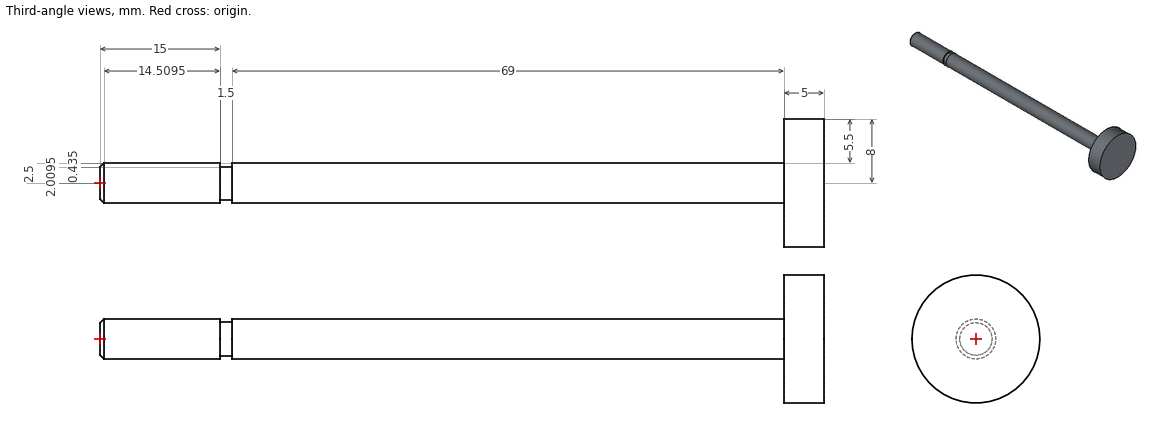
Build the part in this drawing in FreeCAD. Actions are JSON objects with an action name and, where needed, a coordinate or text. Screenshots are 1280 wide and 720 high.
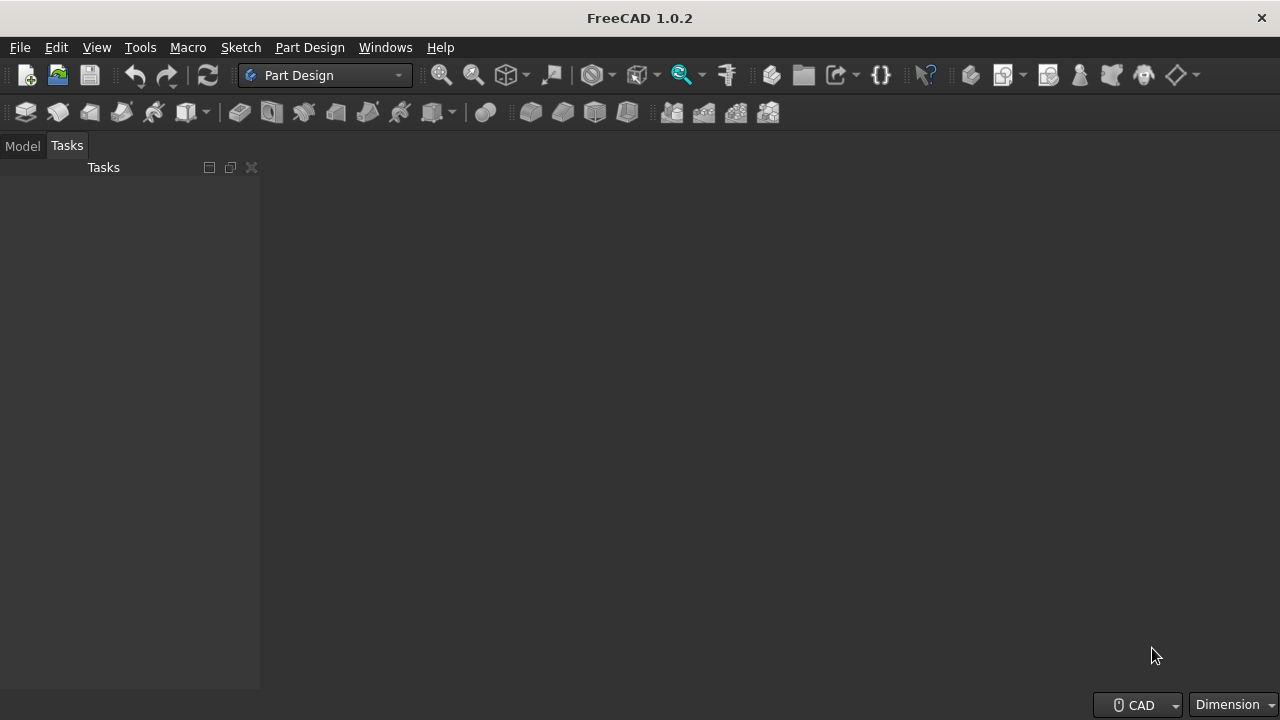
{"action": "left_click", "coordinate": [26, 76]}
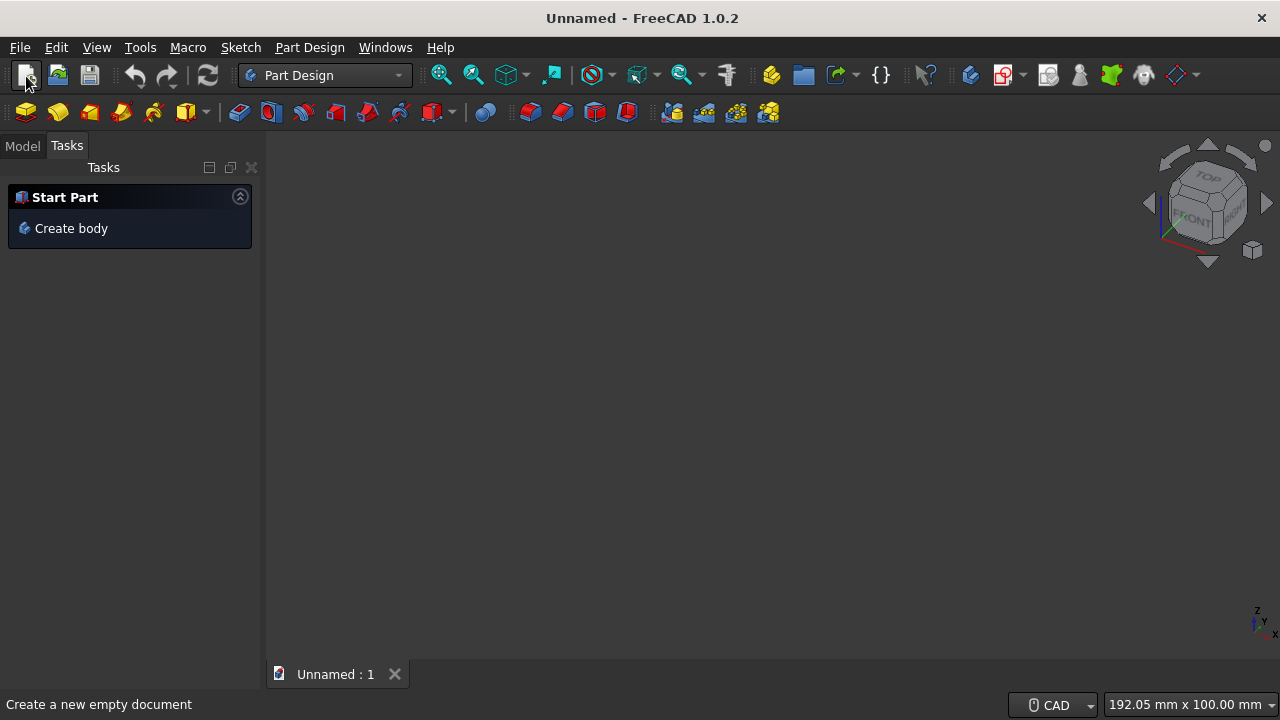
{"action": "left_click", "coordinate": [1004, 76]}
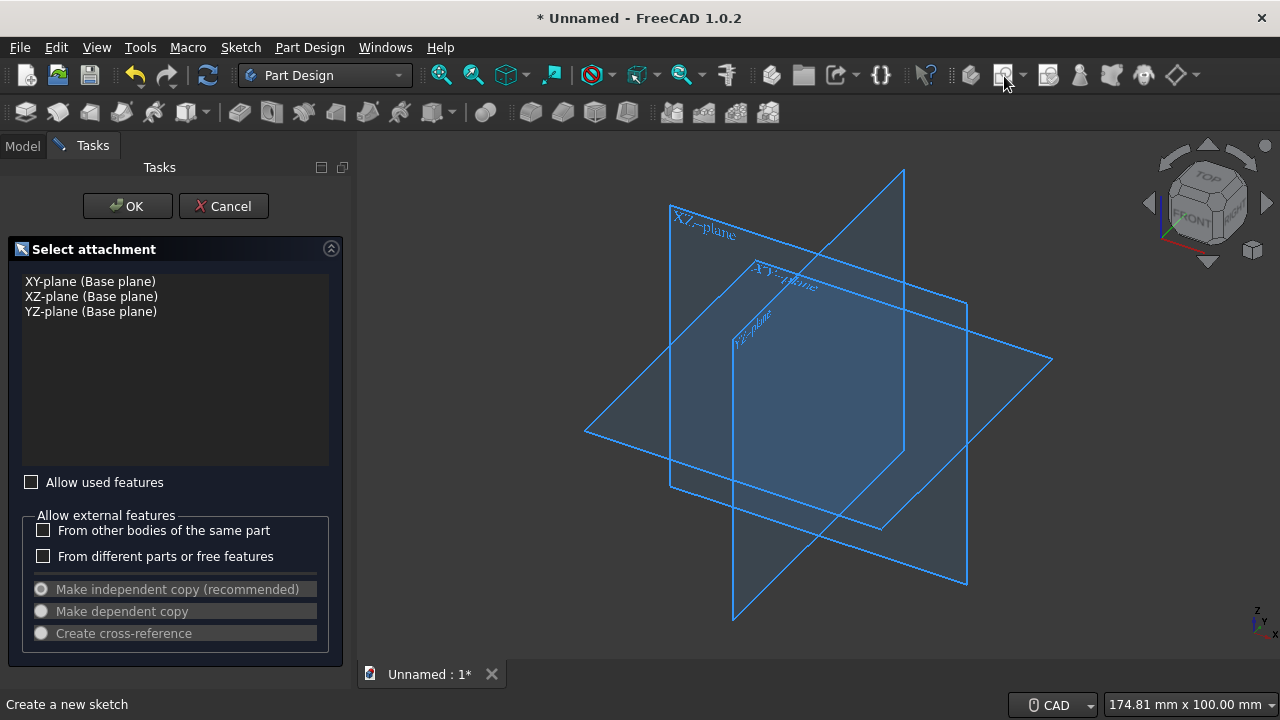
{"action": "left_click", "coordinate": [82, 282]}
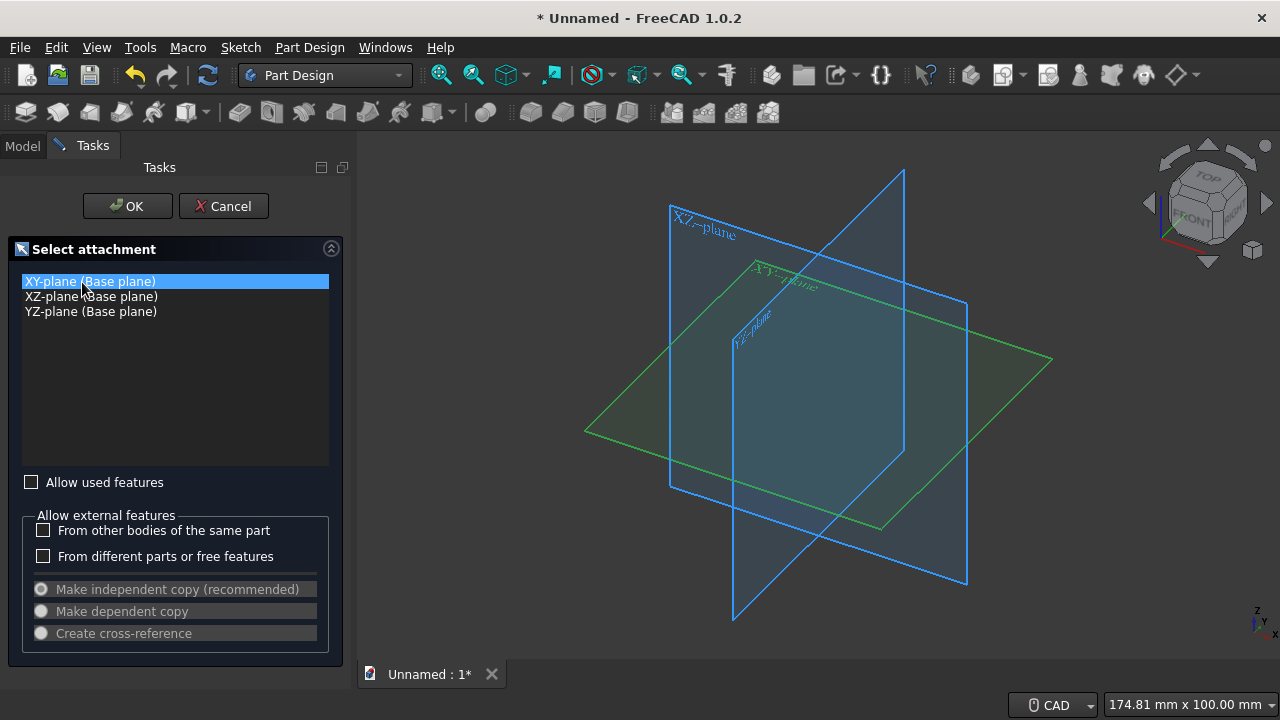
{"action": "left_click", "coordinate": [128, 206]}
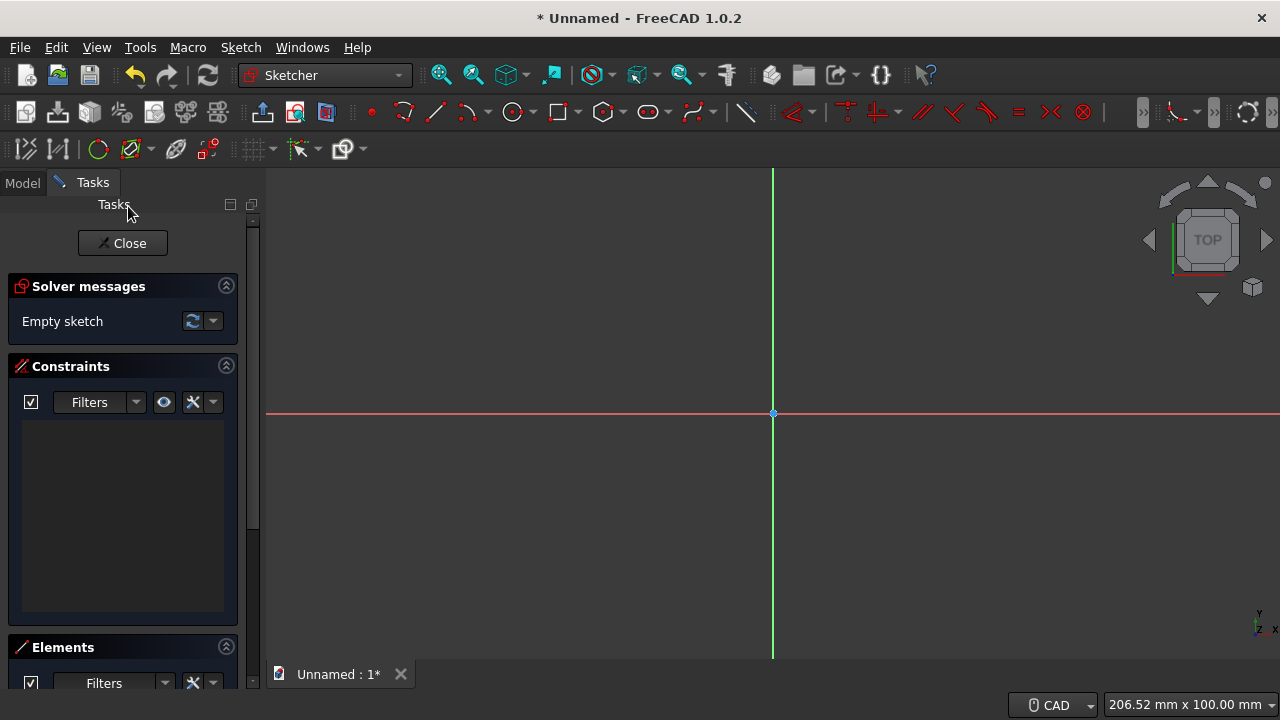
{"action": "scroll", "coordinate": [294, 502], "scroll_direction": "down", "scroll_amount": 1}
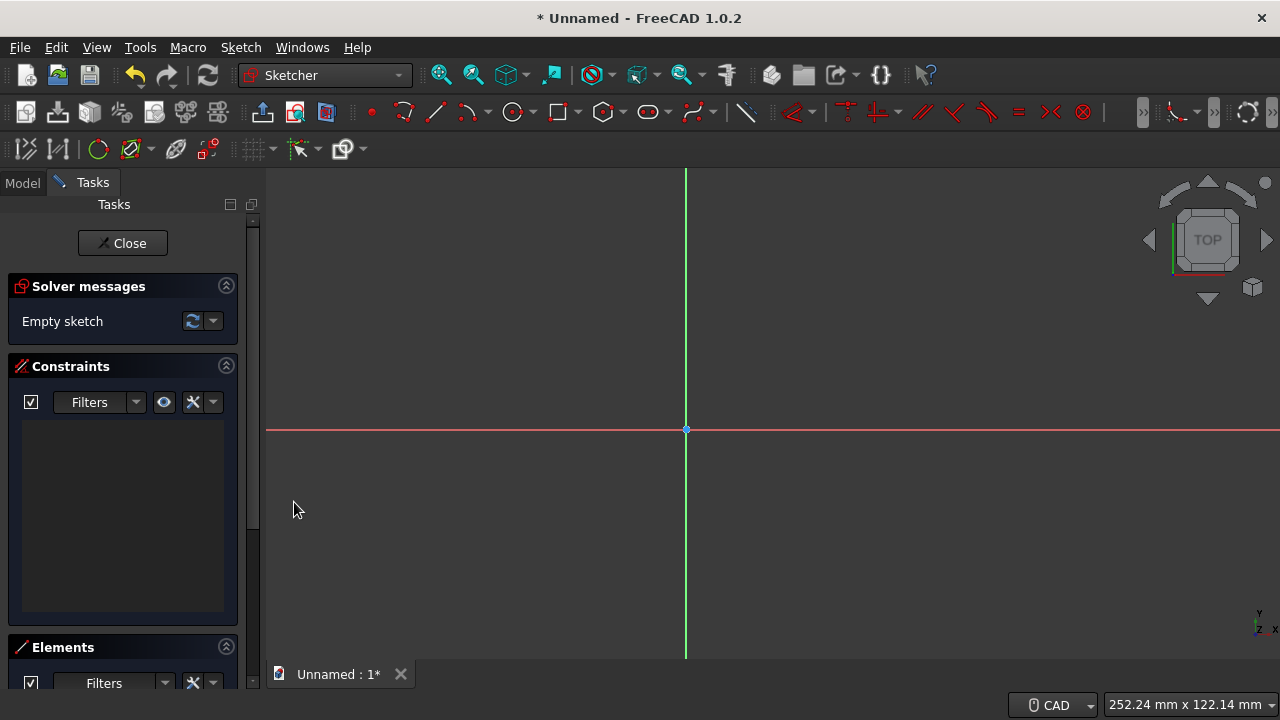
{"action": "scroll", "coordinate": [1115, 414], "scroll_direction": "up", "scroll_amount": 2}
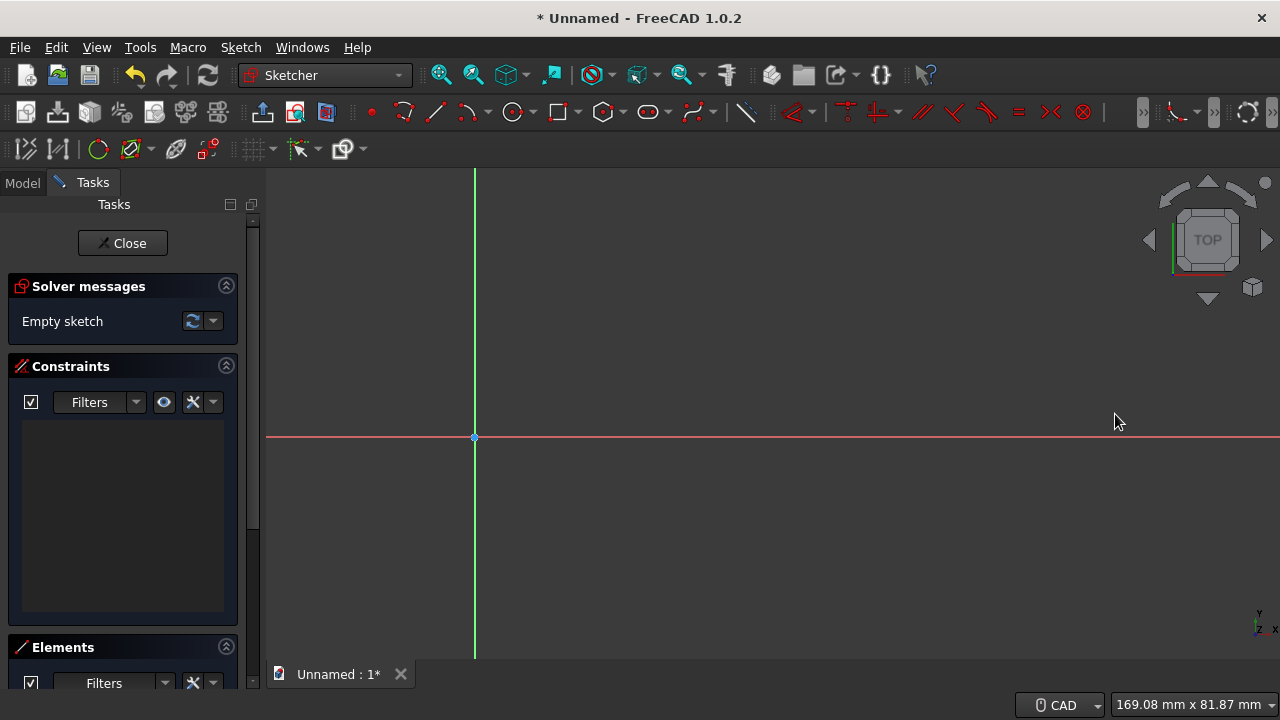
{"action": "left_click", "coordinate": [404, 112]}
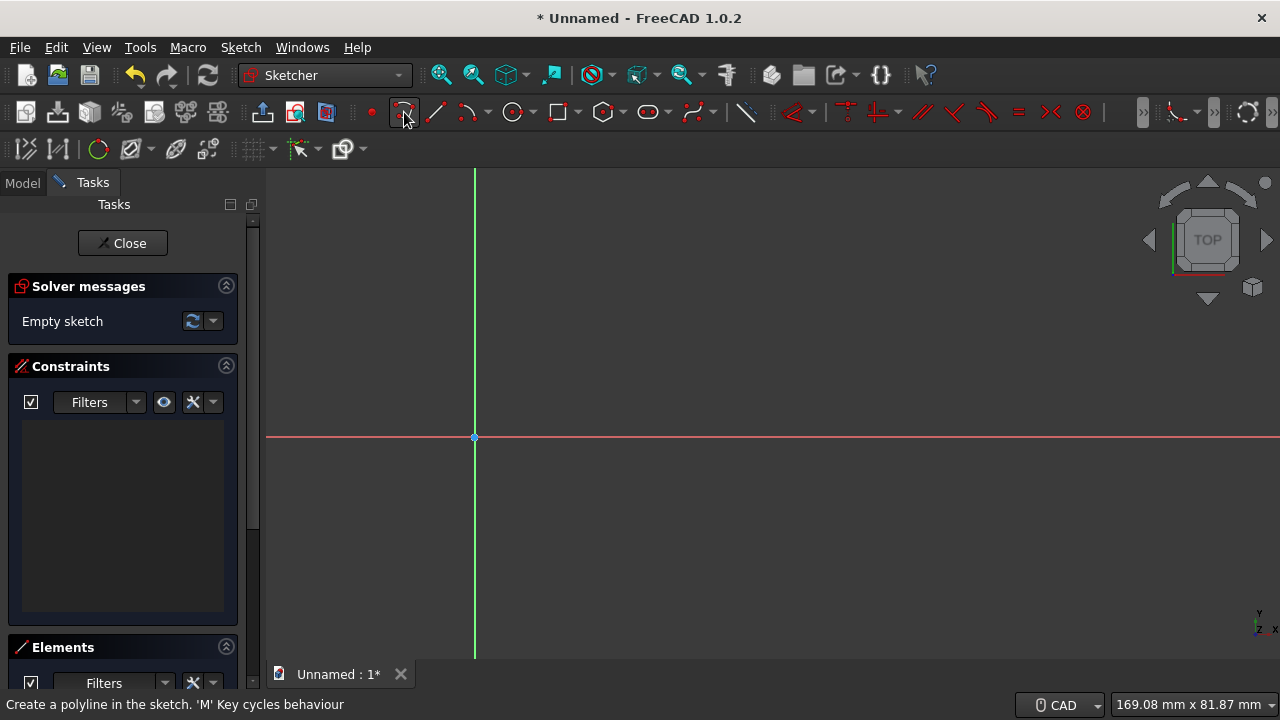
{"action": "left_click", "coordinate": [475, 437]}
{"action": "left_click", "coordinate": [1018, 428]}
{"action": "left_click", "coordinate": [1018, 389]}
{"action": "left_click", "coordinate": [988, 389]}
{"action": "left_click", "coordinate": [988, 422]}
{"action": "left_click", "coordinate": [574, 422]}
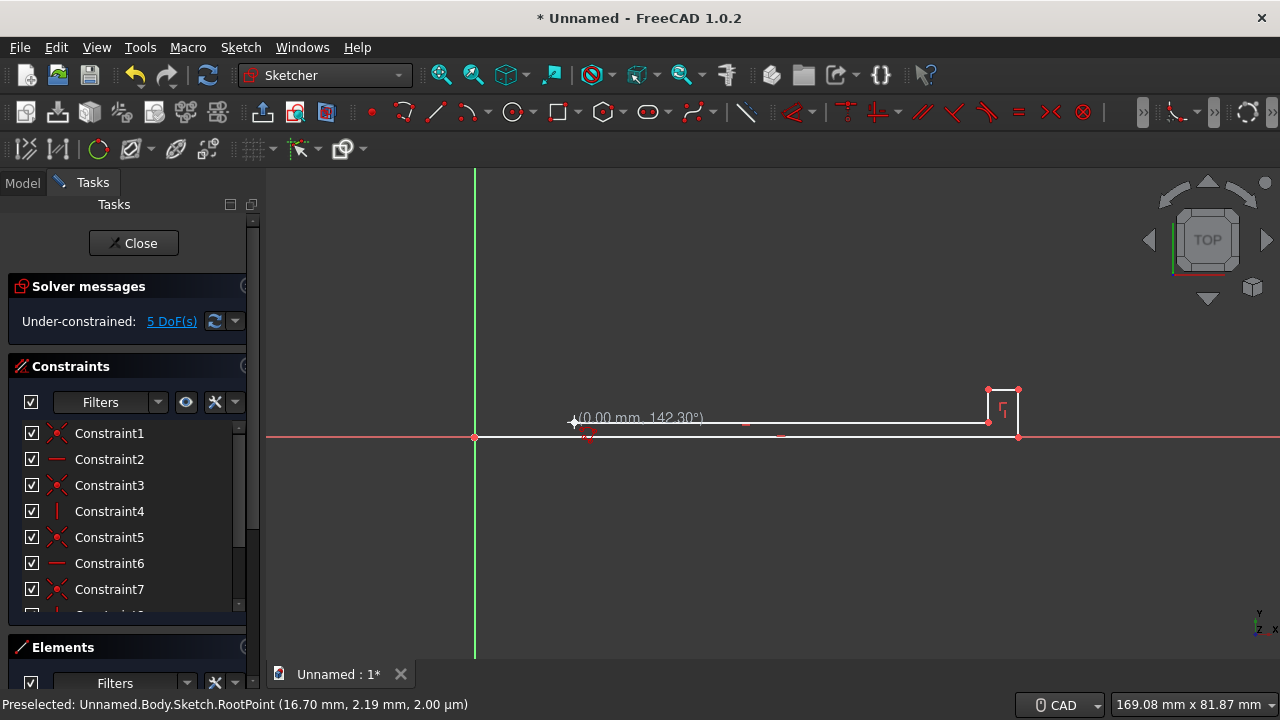
{"action": "scroll", "coordinate": [574, 425], "scroll_direction": "up", "scroll_amount": 10}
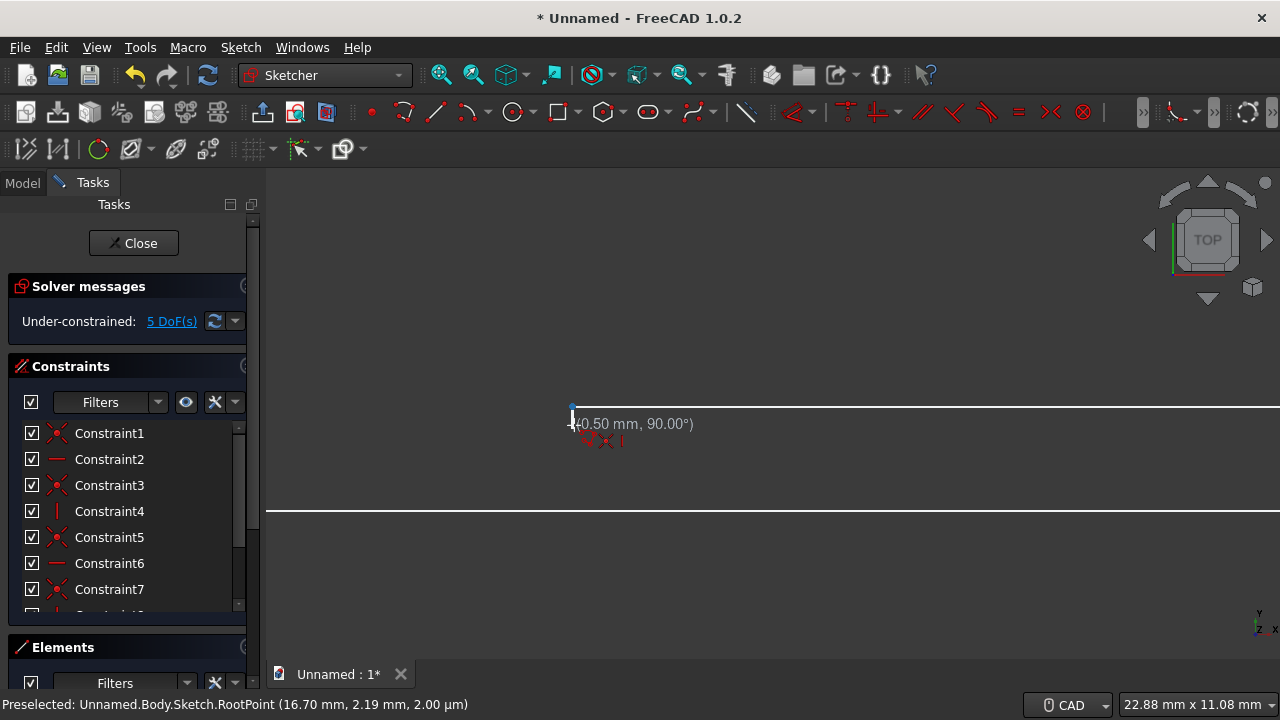
{"action": "left_click", "coordinate": [572, 420]}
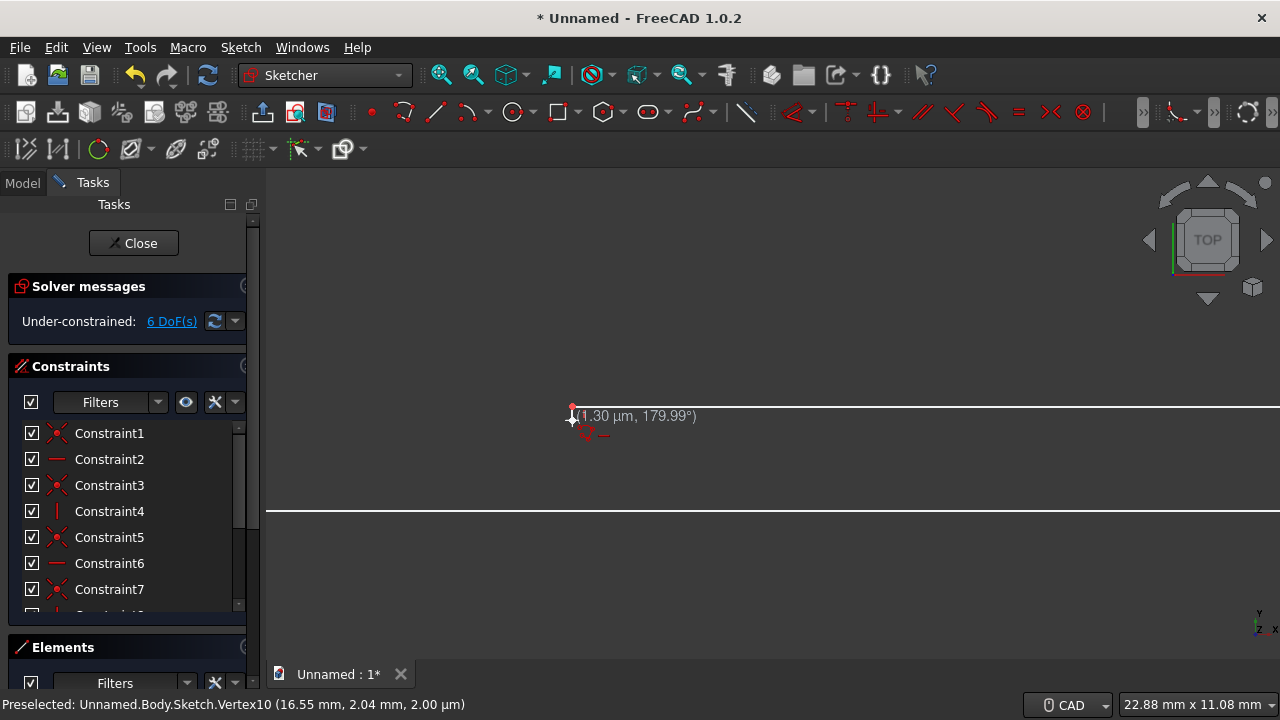
{"action": "scroll", "coordinate": [526, 426], "scroll_direction": "down", "scroll_amount": 10}